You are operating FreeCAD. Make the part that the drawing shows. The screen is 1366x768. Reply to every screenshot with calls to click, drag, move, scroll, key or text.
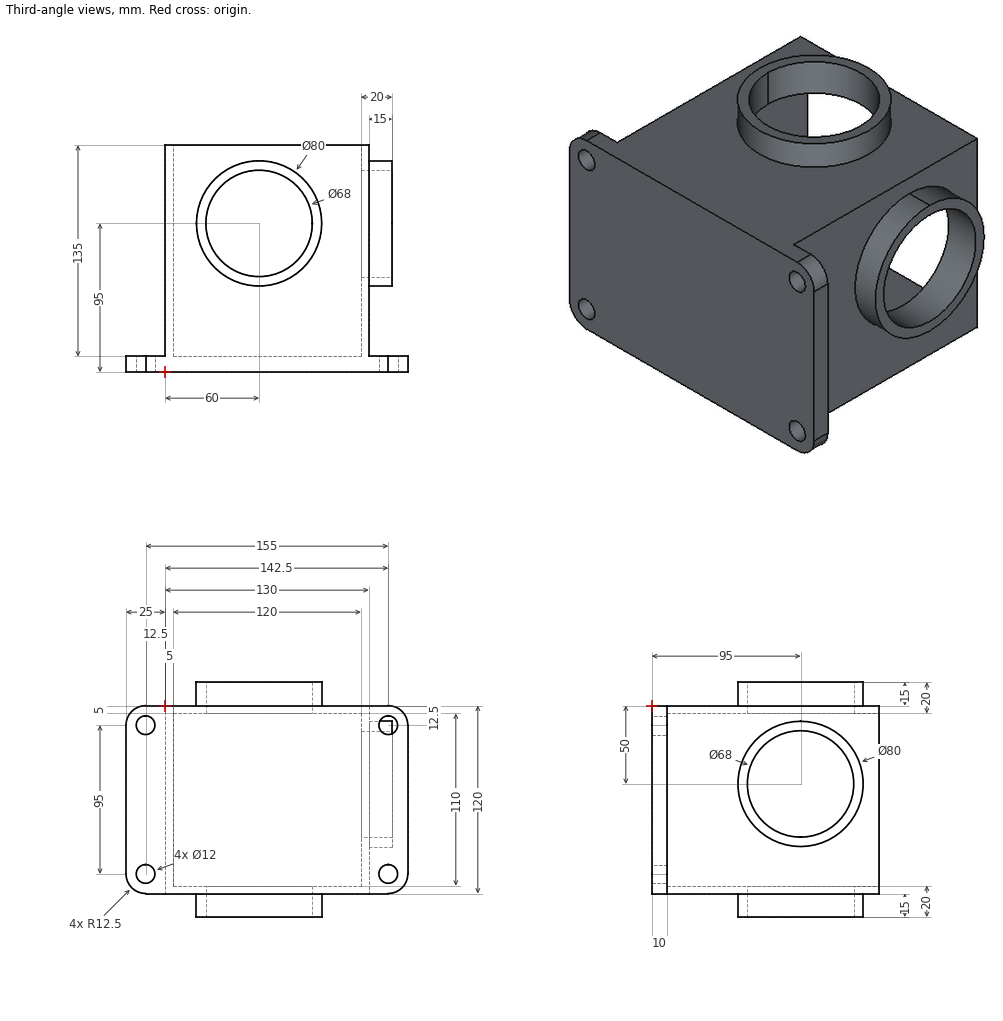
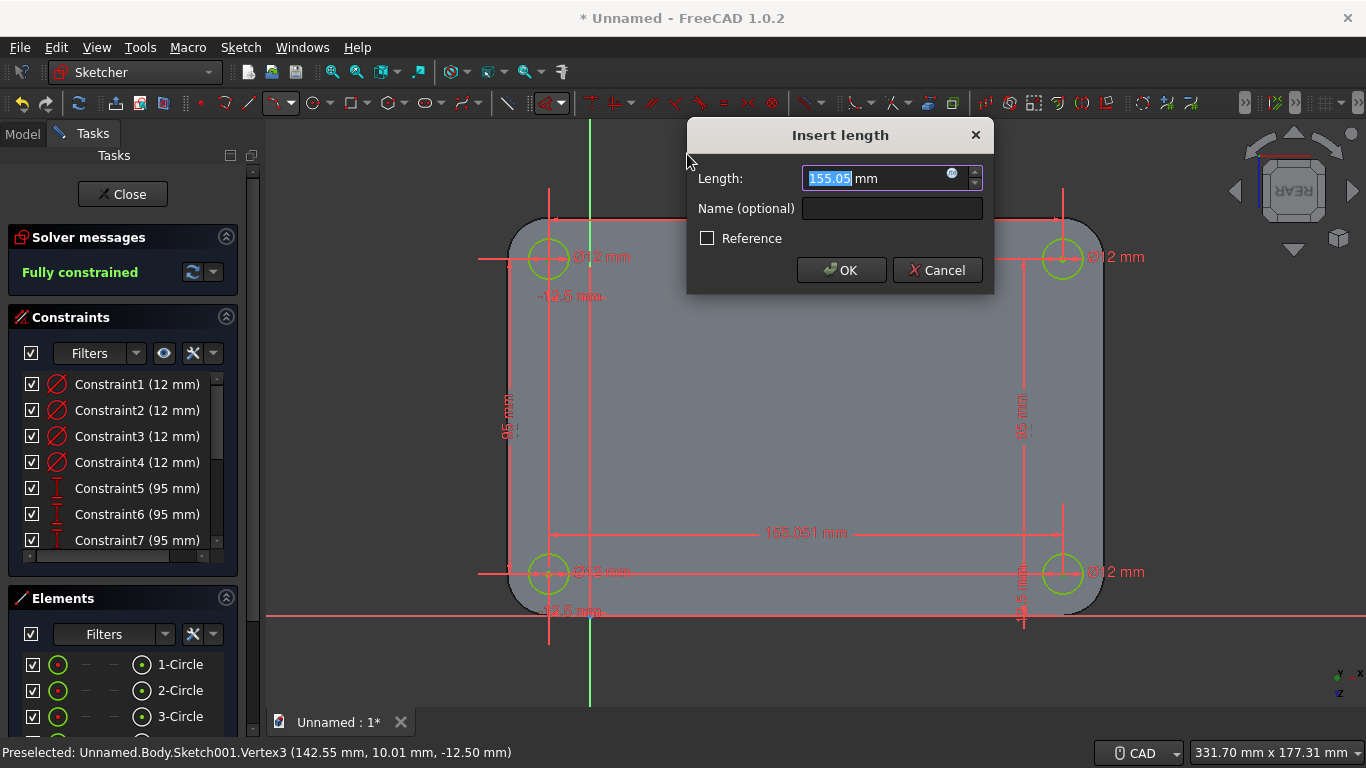
text(155)
key(Return)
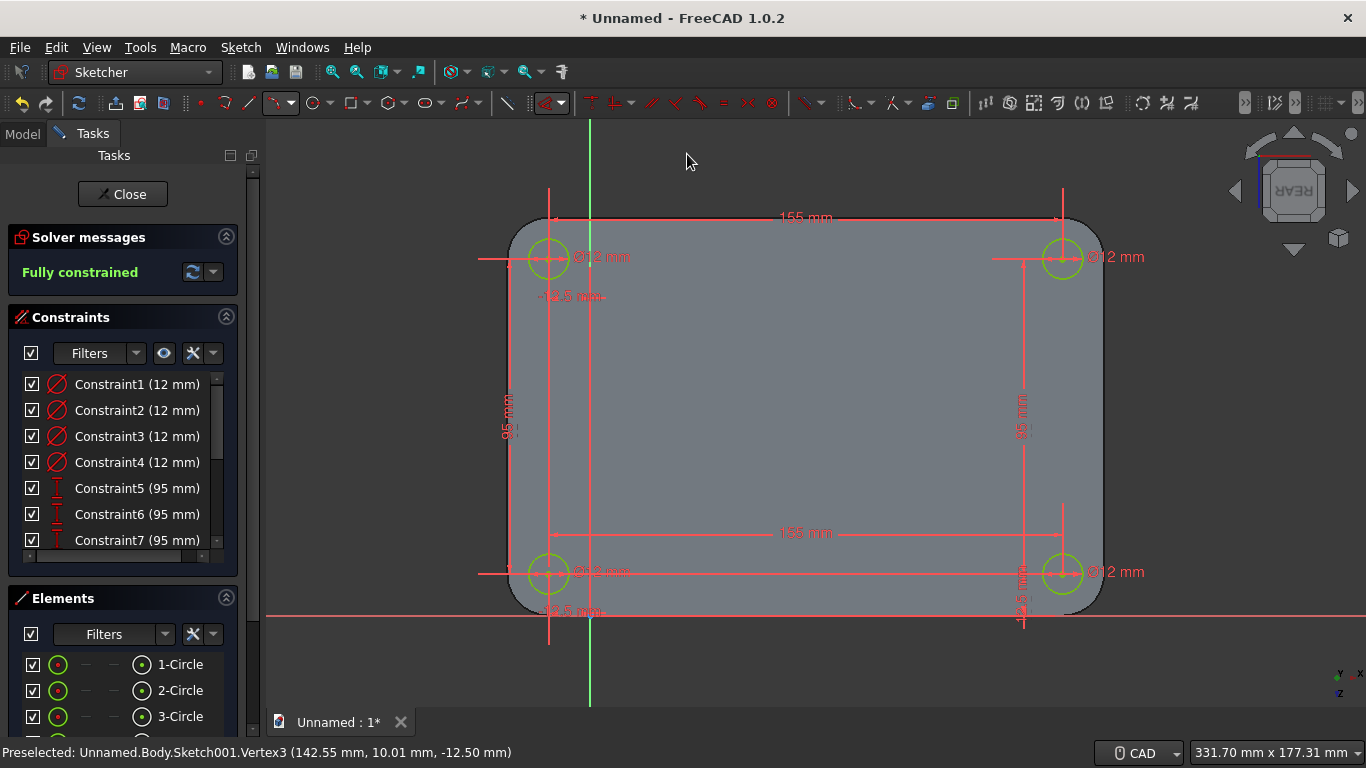
click(123, 194)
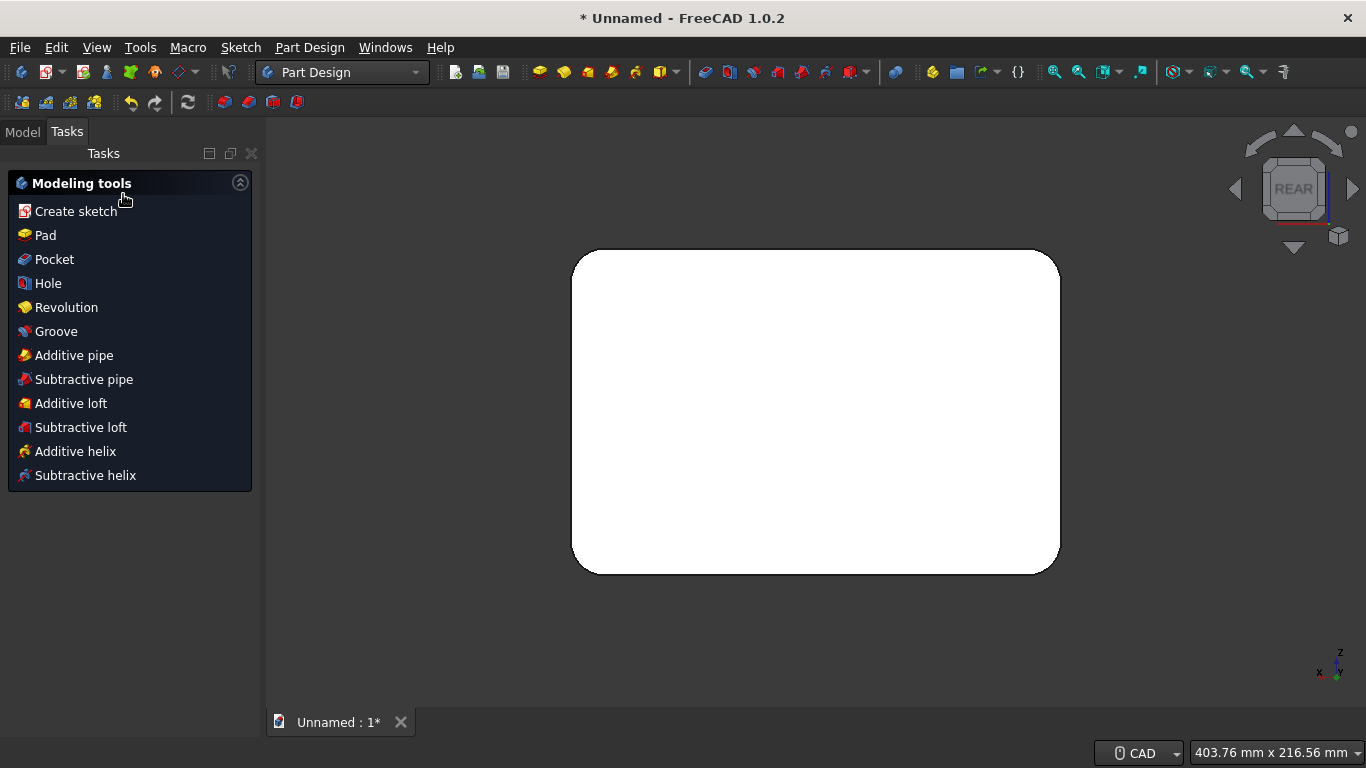
click(706, 72)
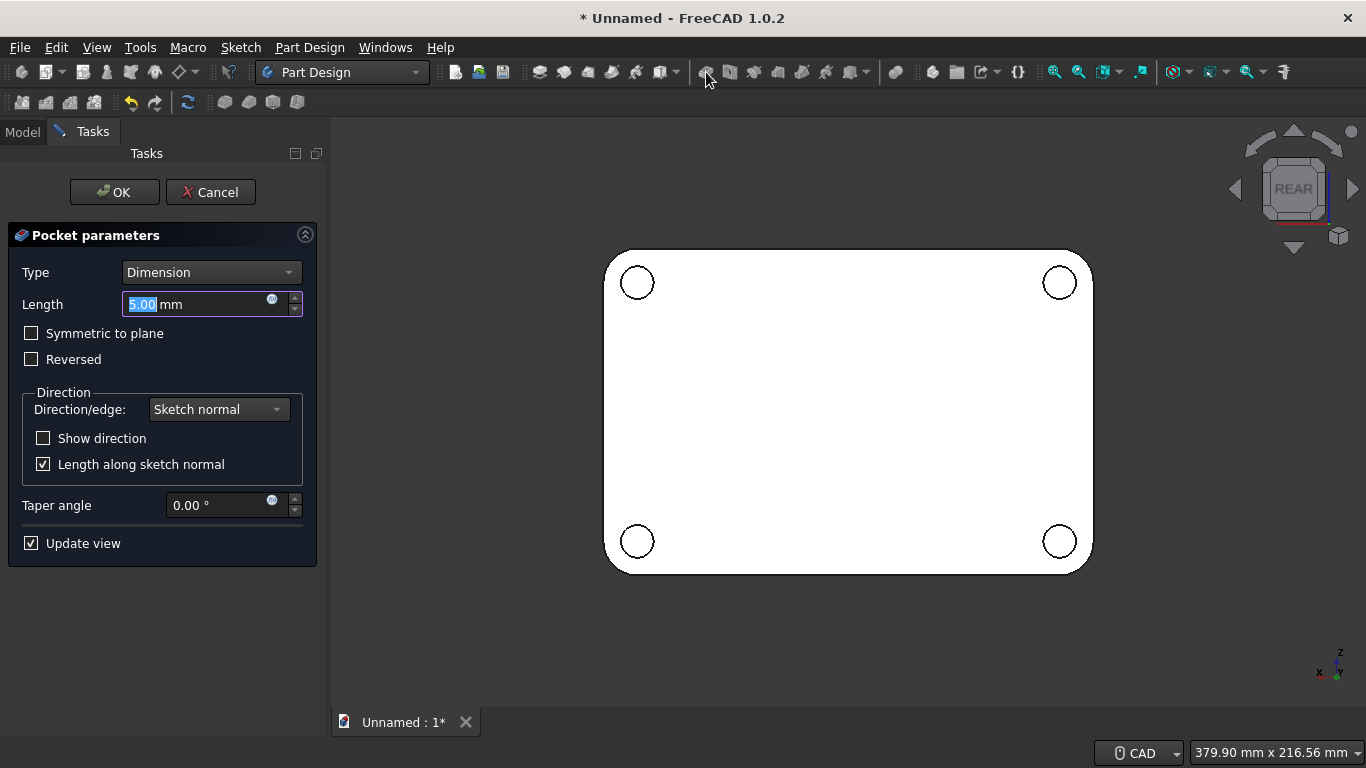
click(212, 272)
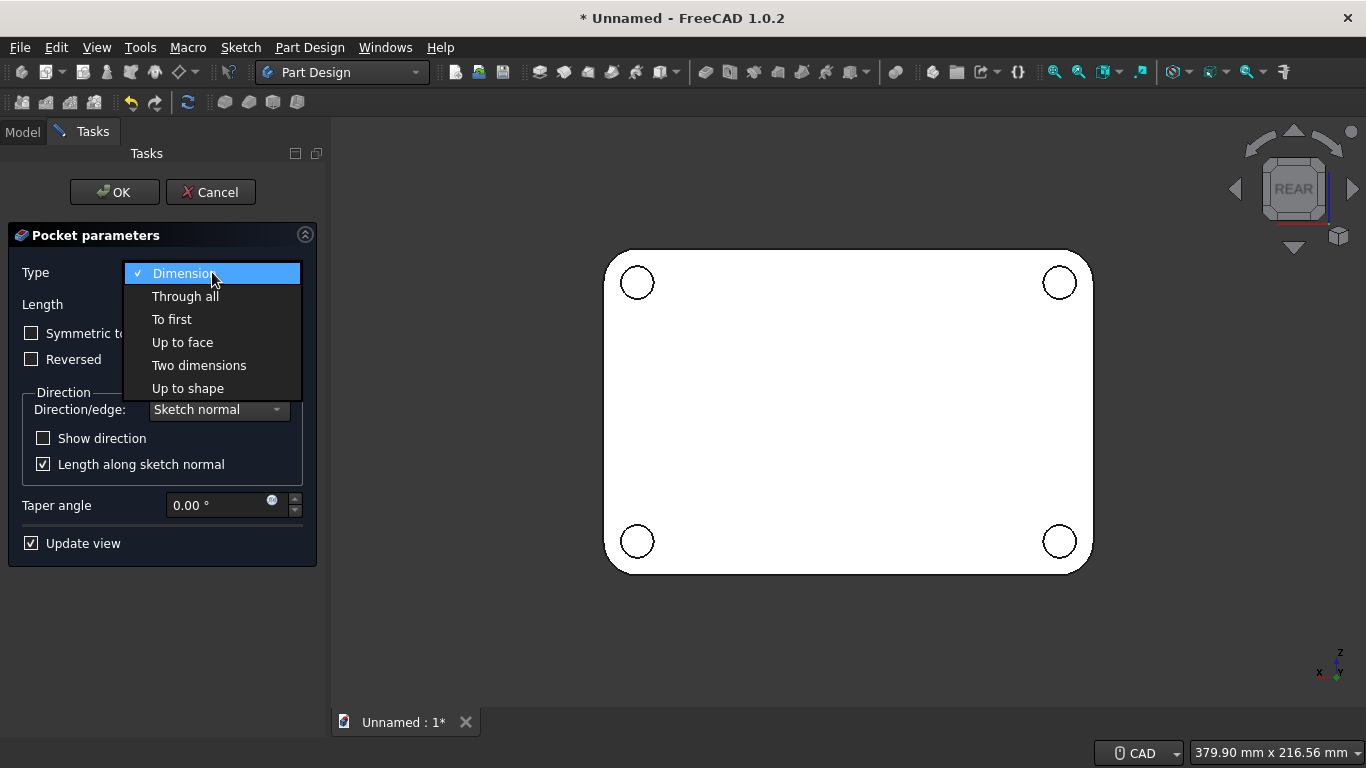
click(212, 296)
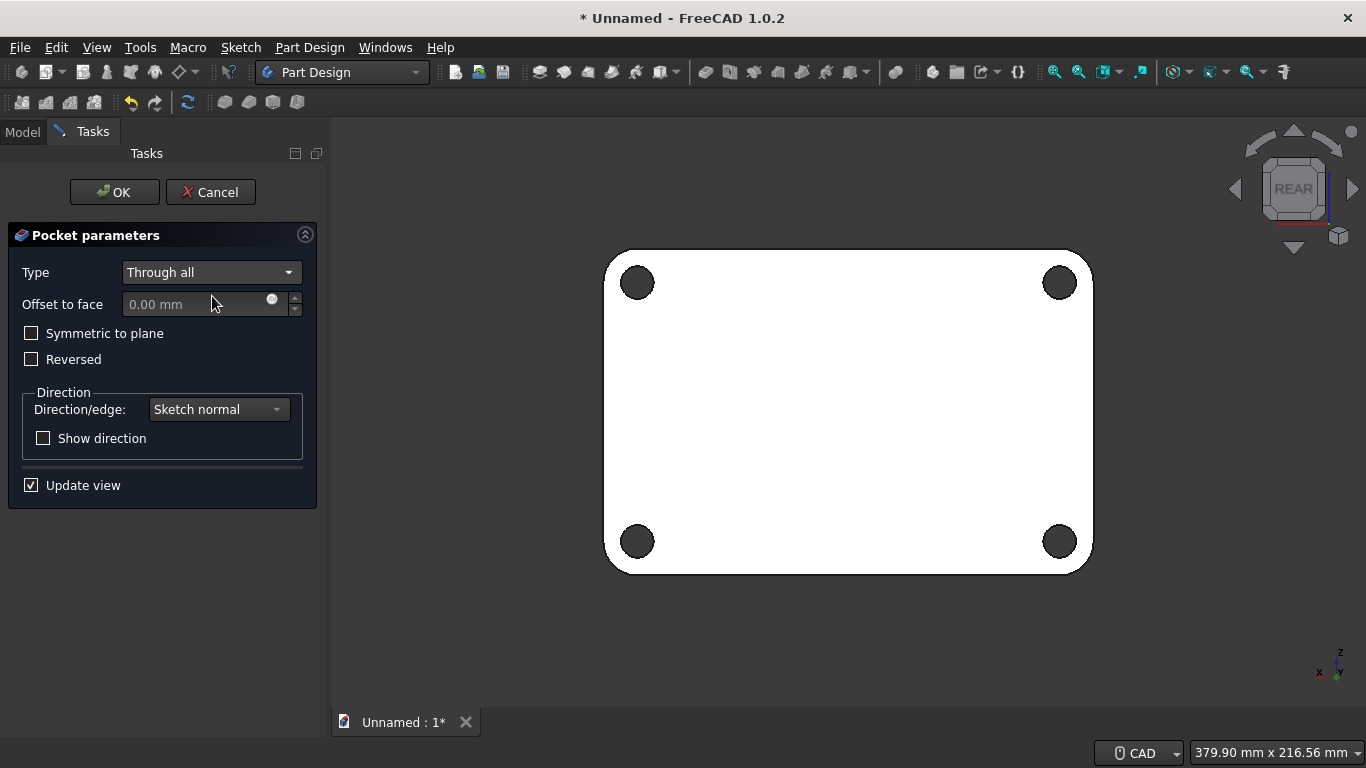
click(115, 192)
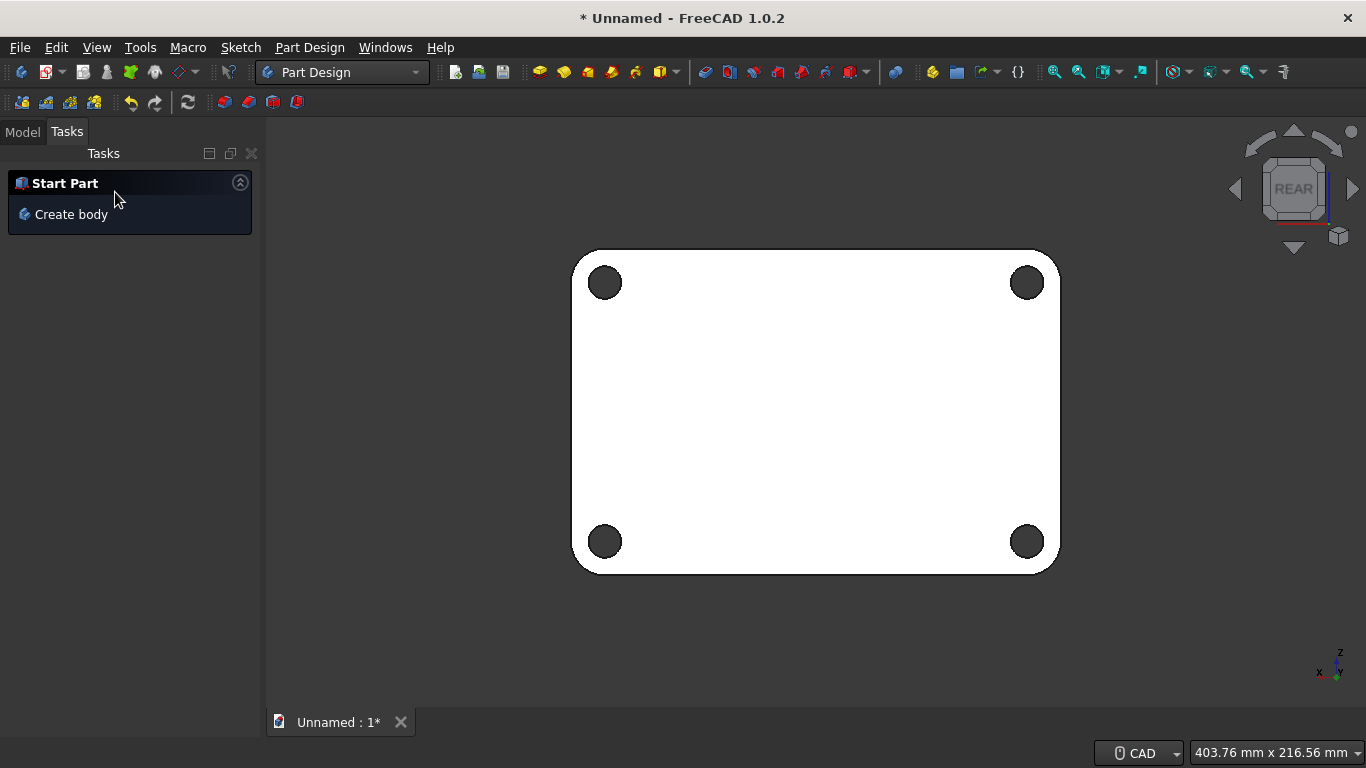
click(746, 411)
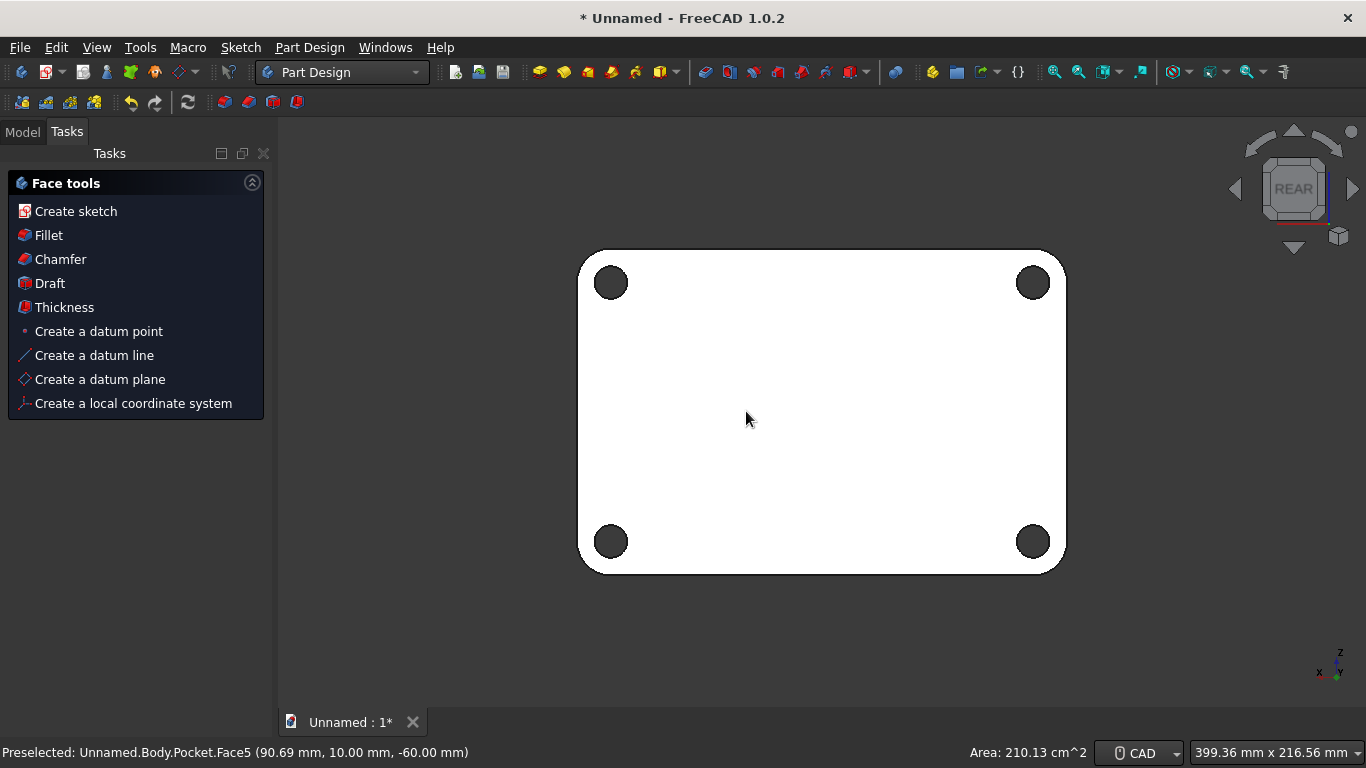
click(46, 72)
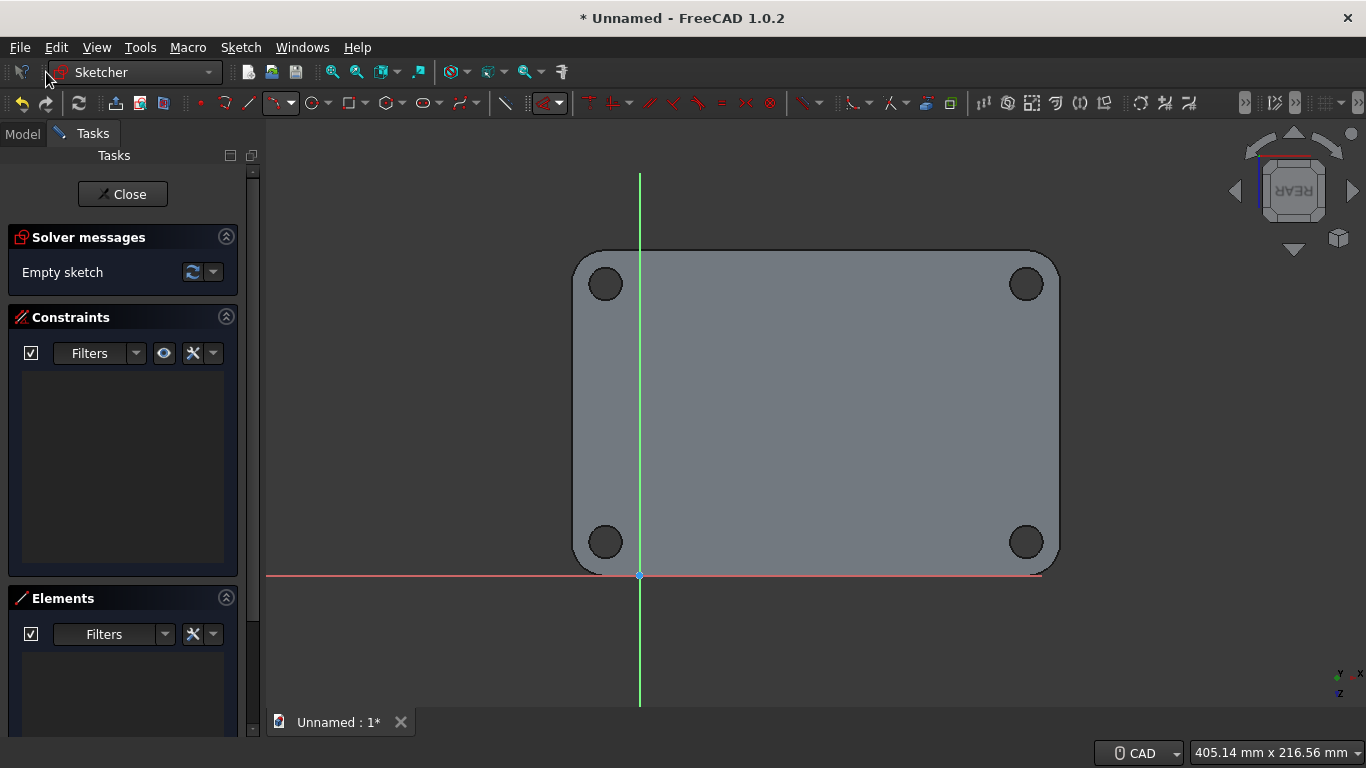
key(g)
key(r)